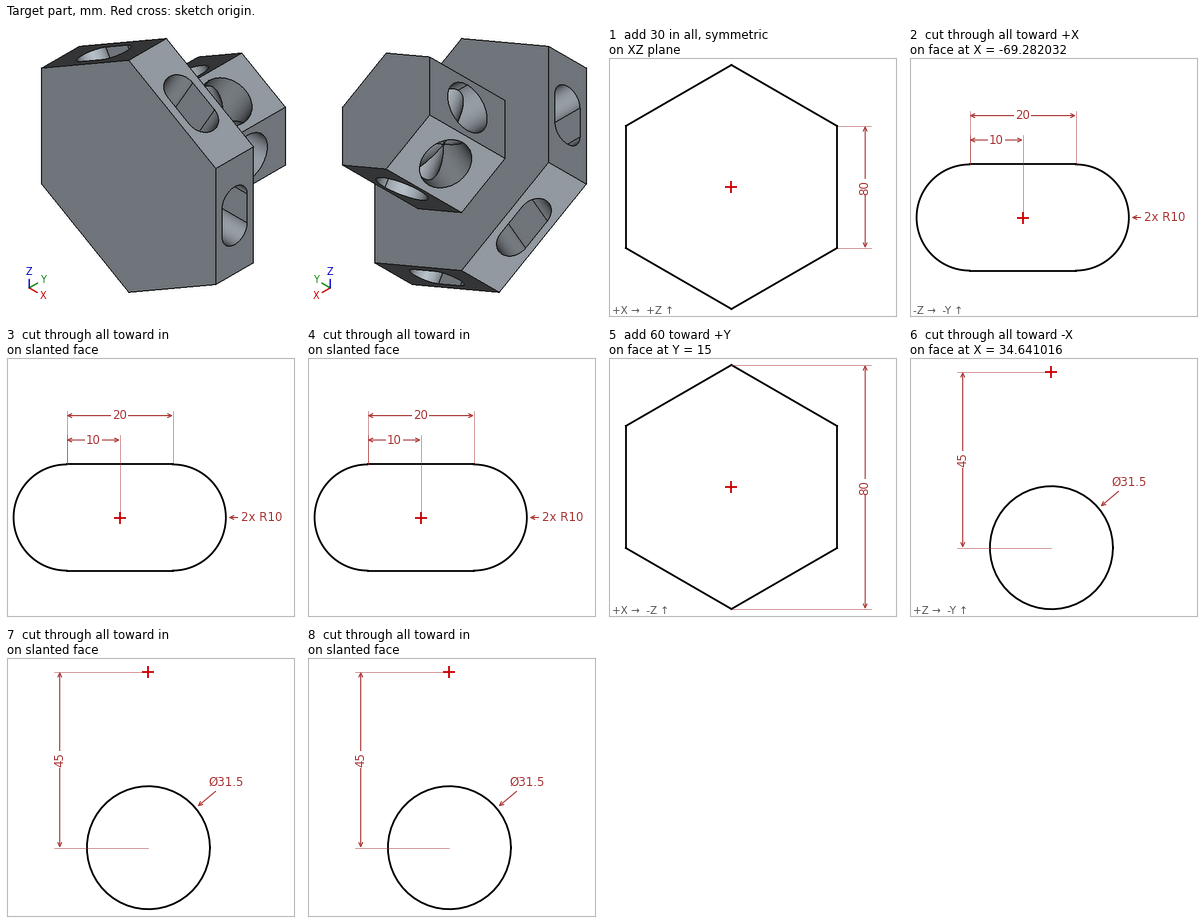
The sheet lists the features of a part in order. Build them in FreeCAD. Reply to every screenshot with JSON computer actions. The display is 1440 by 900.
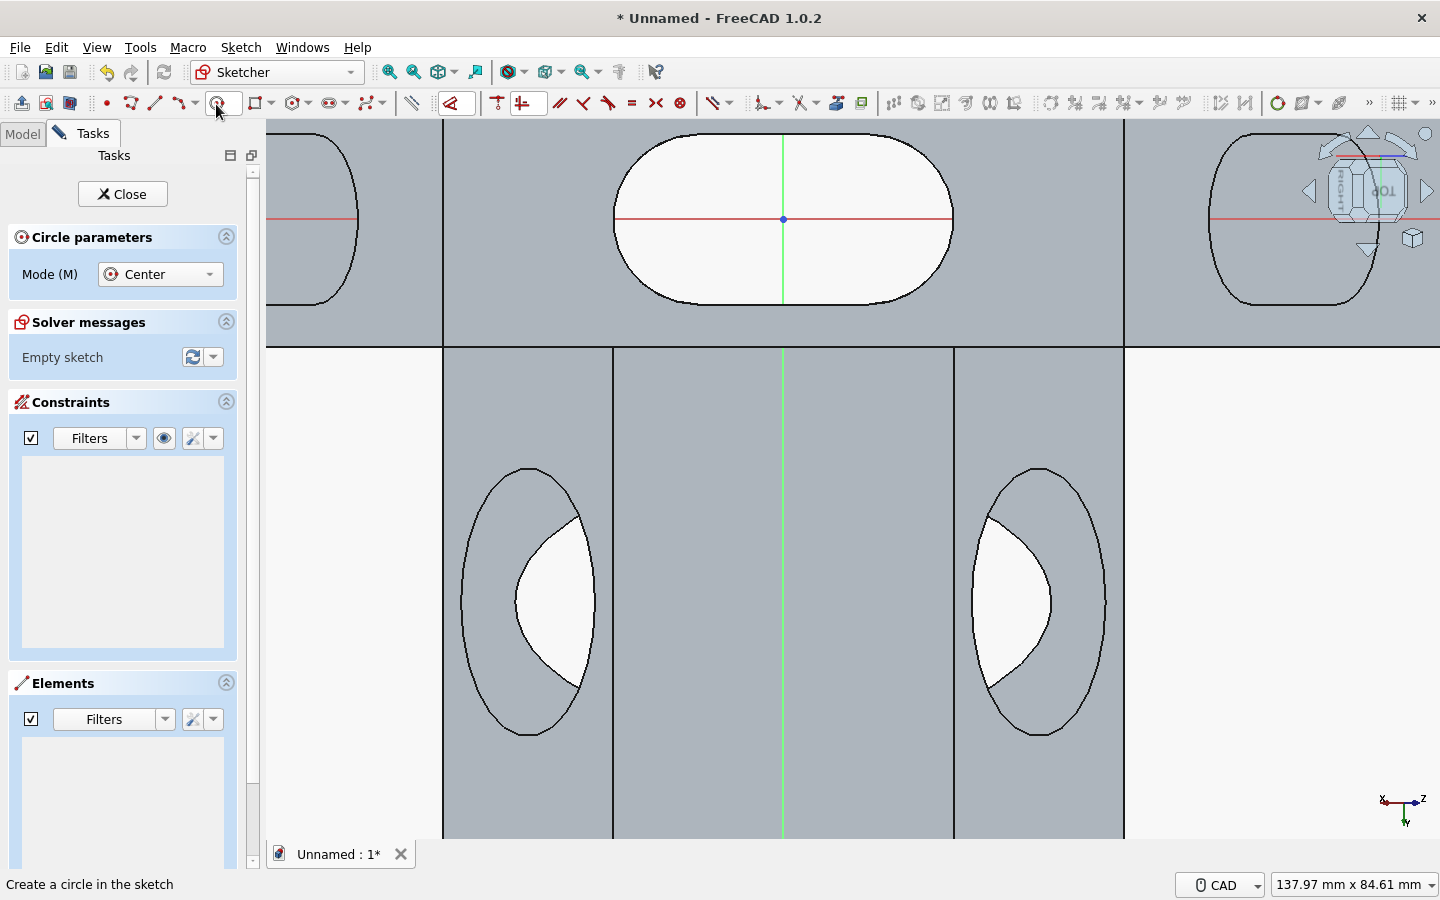
{"action": "left_click", "coordinate": [783, 602]}
{"action": "mouse_move", "coordinate": [878, 508]}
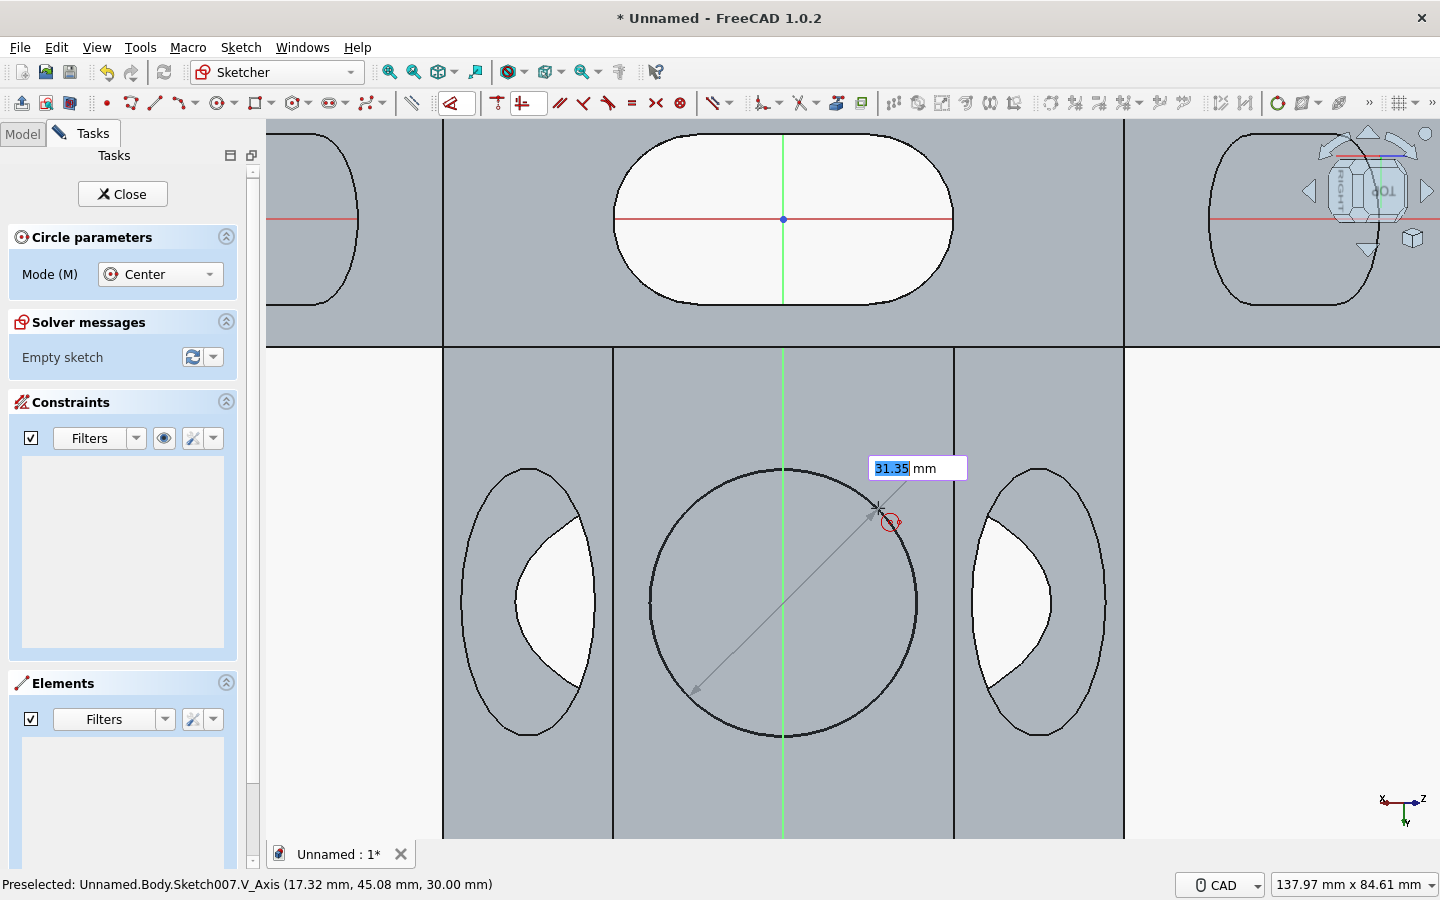
{"action": "type", "text": "31.5"}
{"action": "key", "text": "Return"}
{"action": "key", "text": "Escape"}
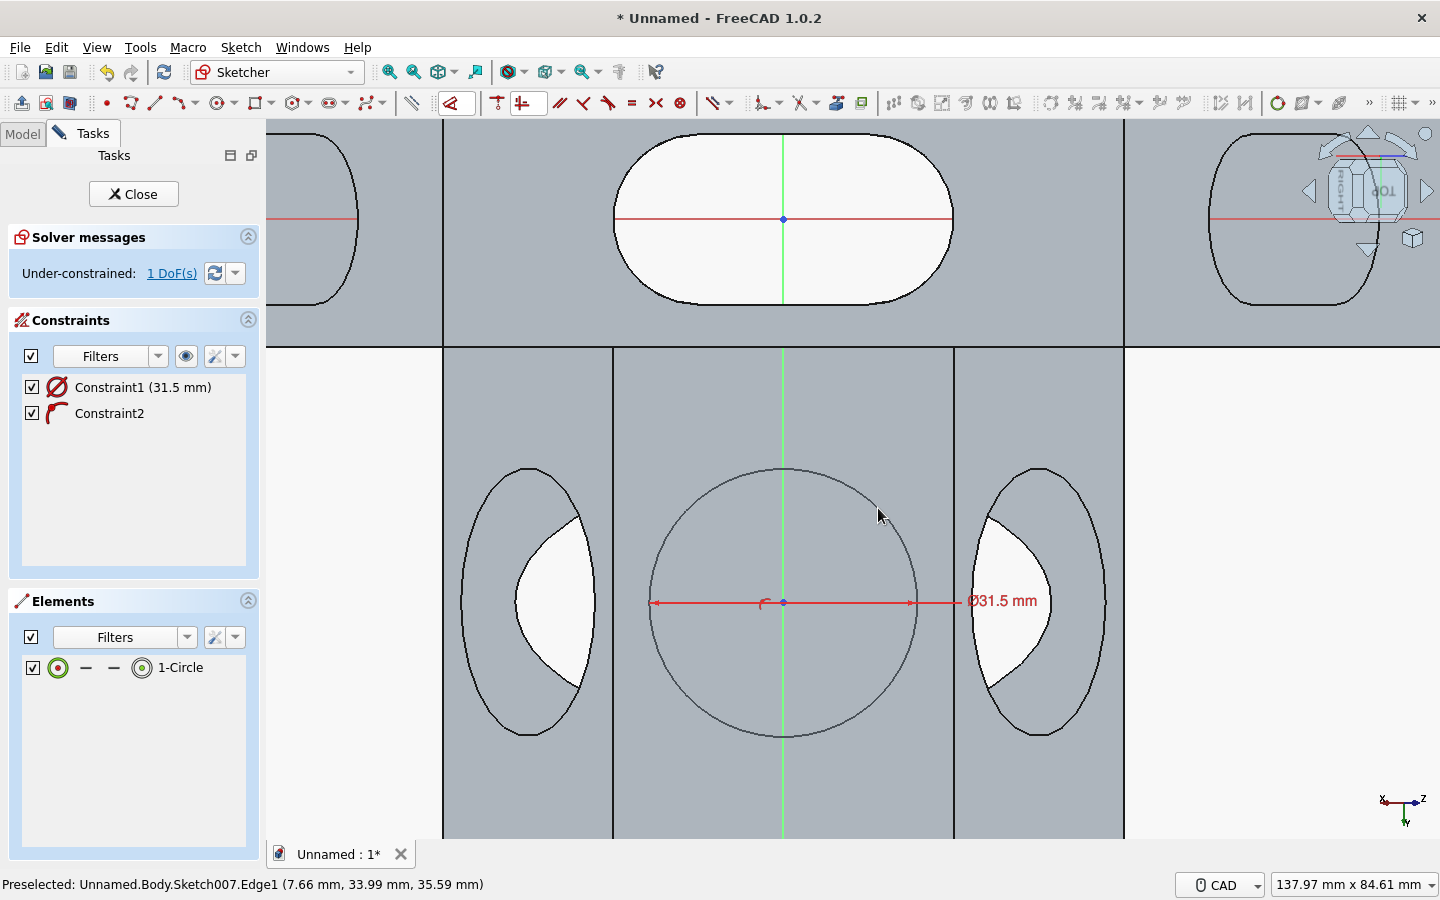
{"action": "left_click", "coordinate": [783, 603]}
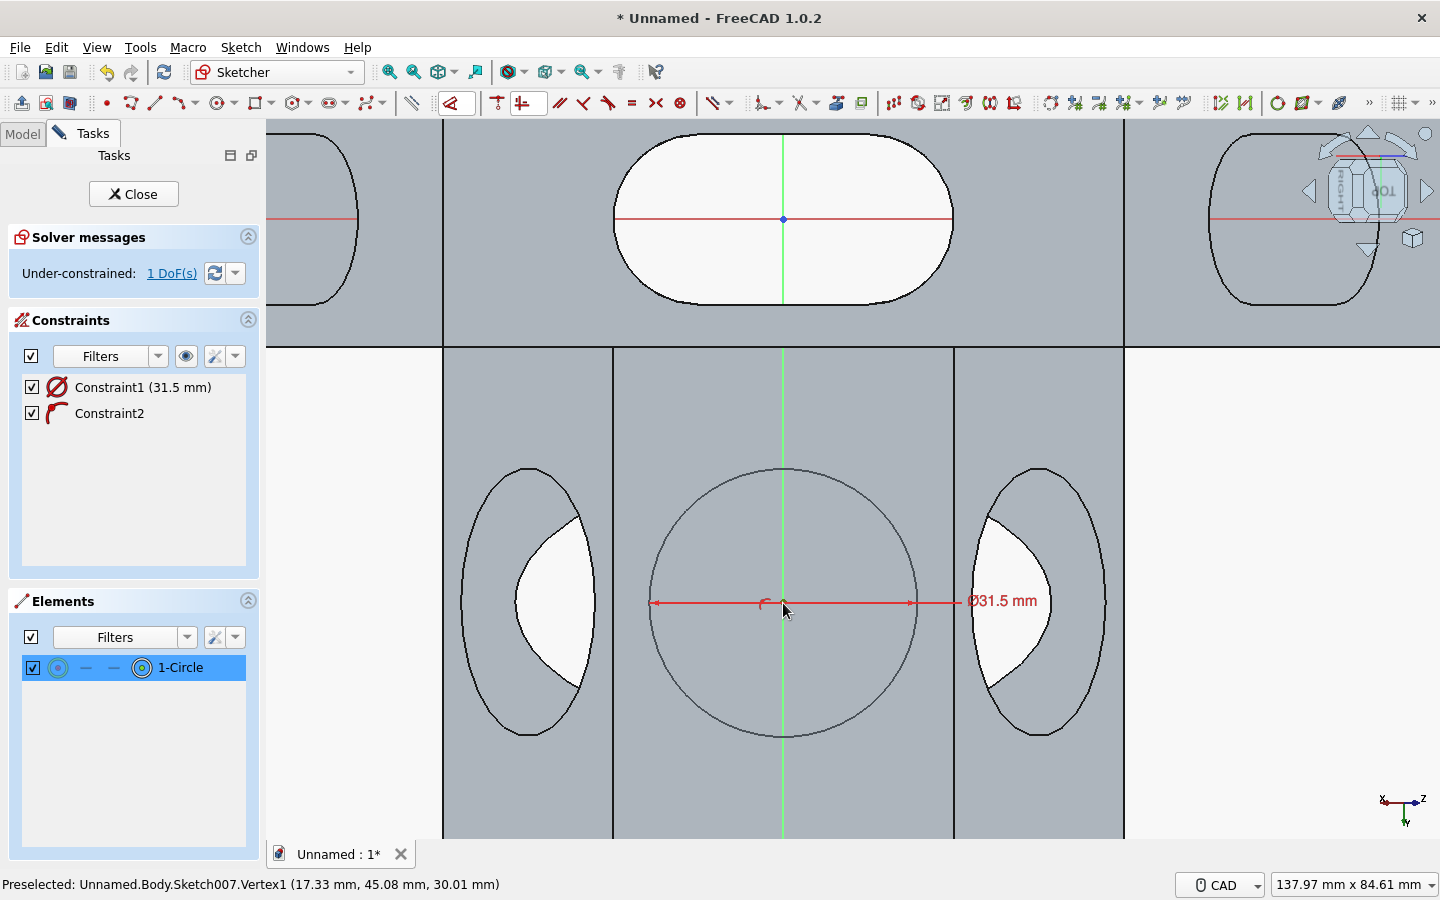
{"action": "key", "text": "i"}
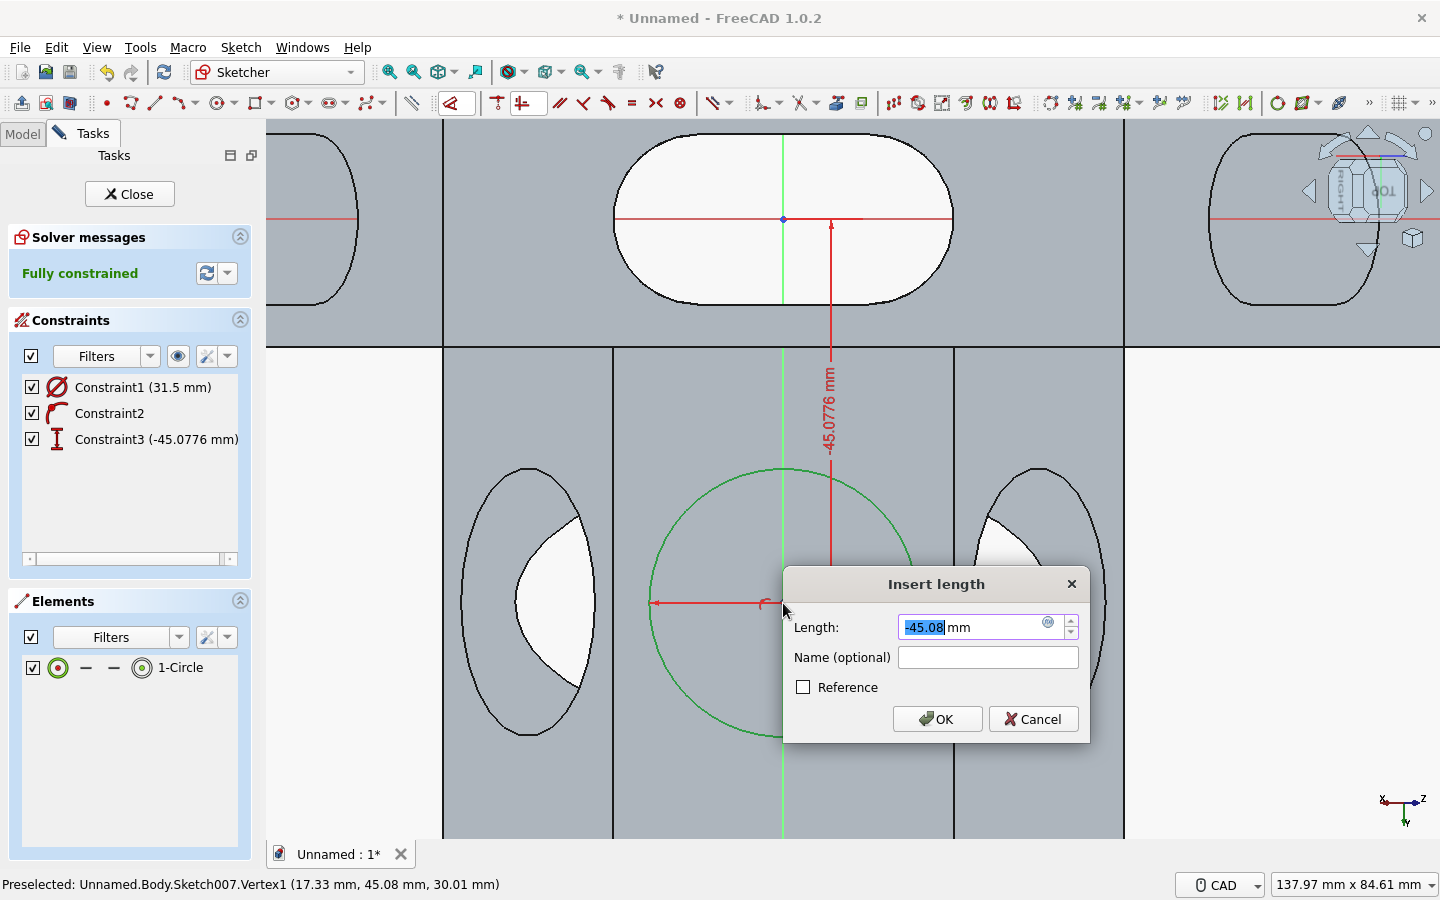
{"action": "type", "text": "-45"}
{"action": "key", "text": "Return"}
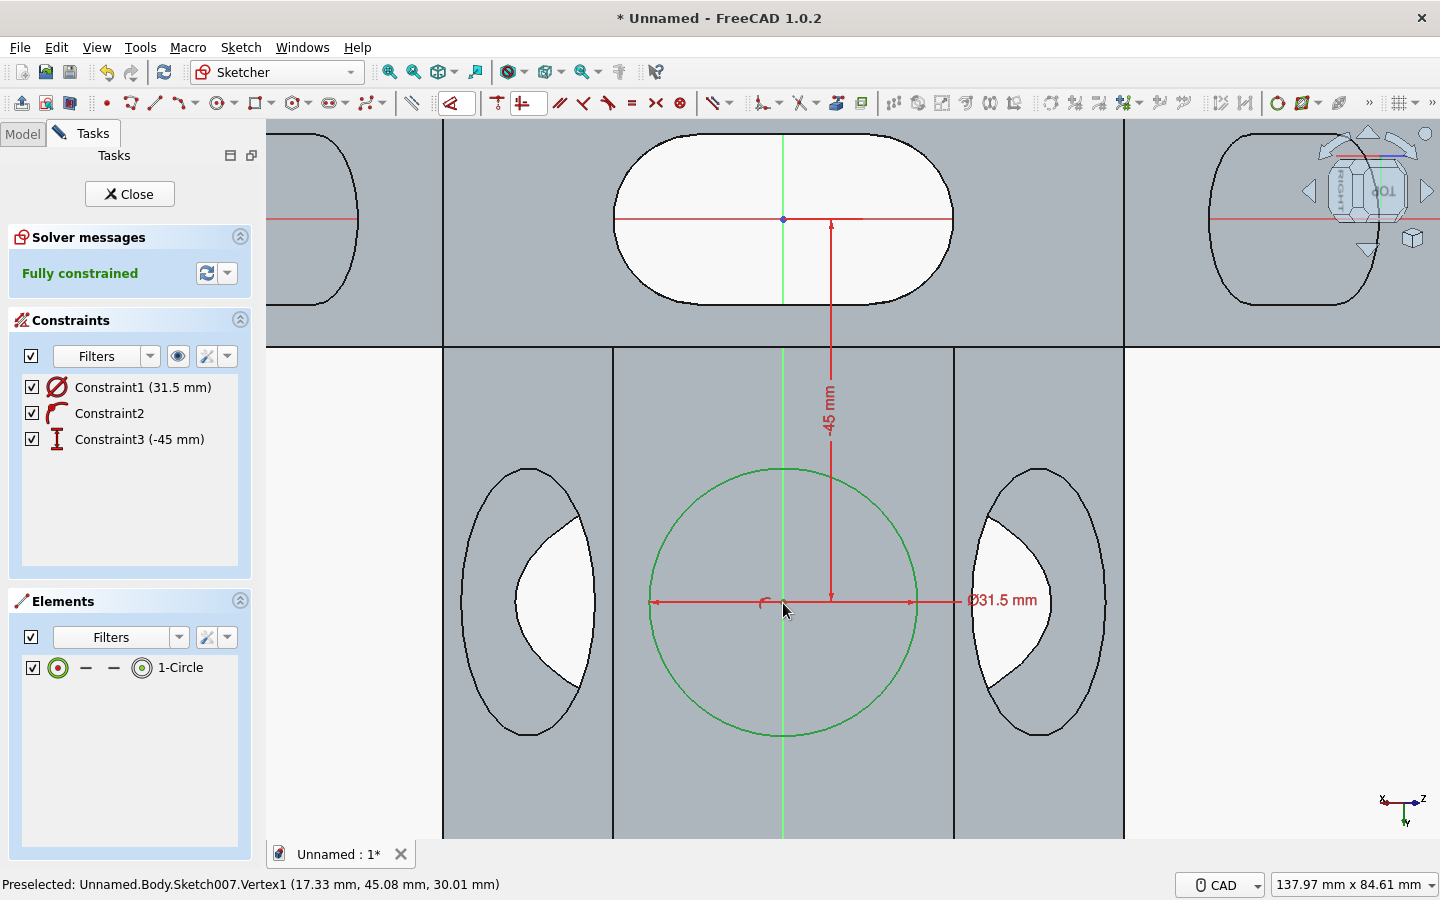
{"action": "left_click", "coordinate": [130, 194]}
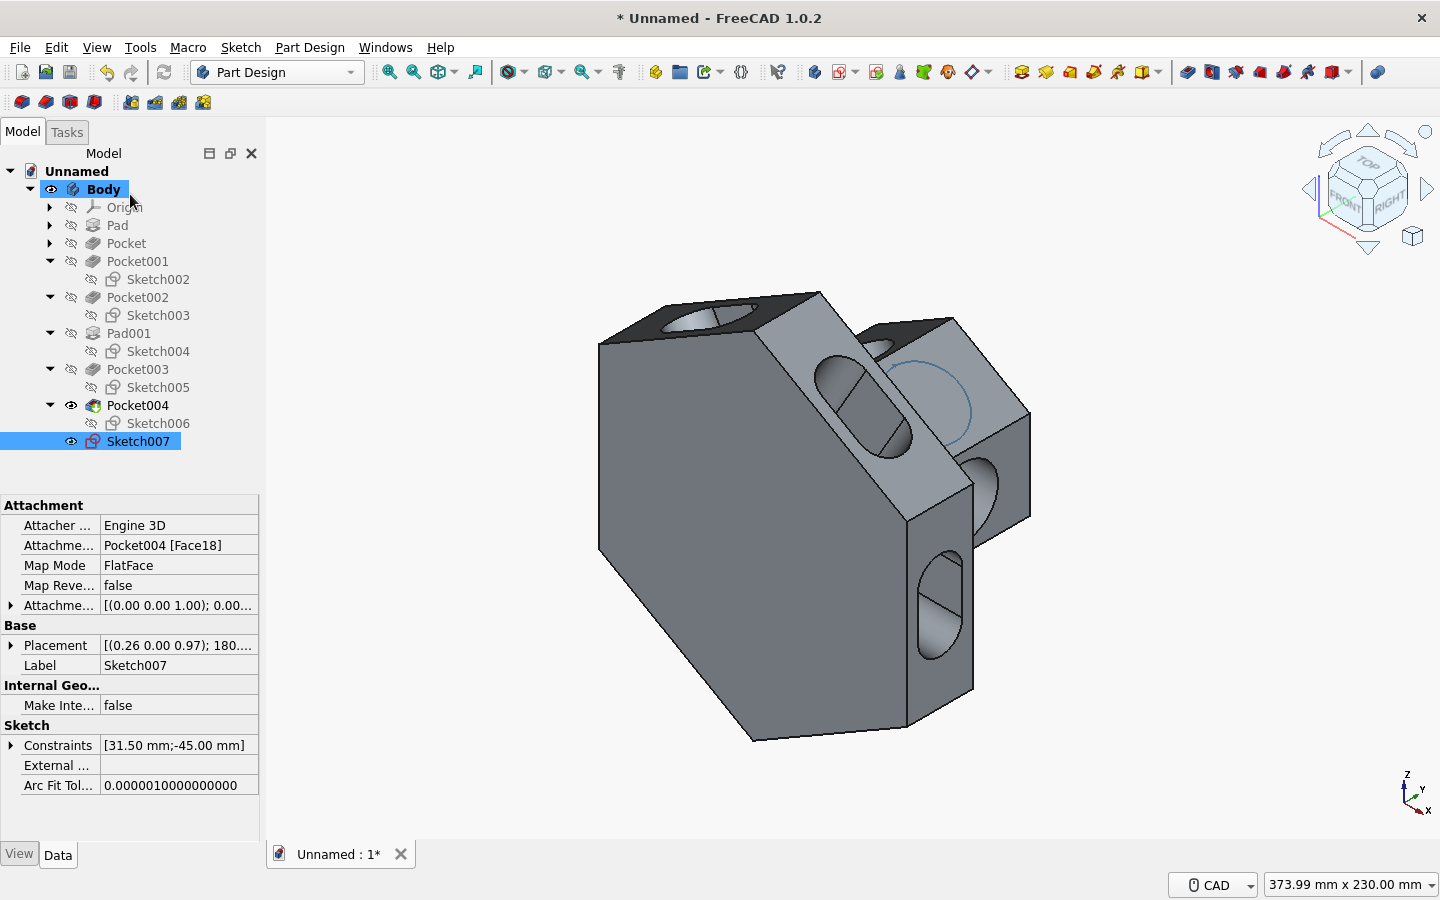
{"action": "left_click", "coordinate": [1188, 72]}